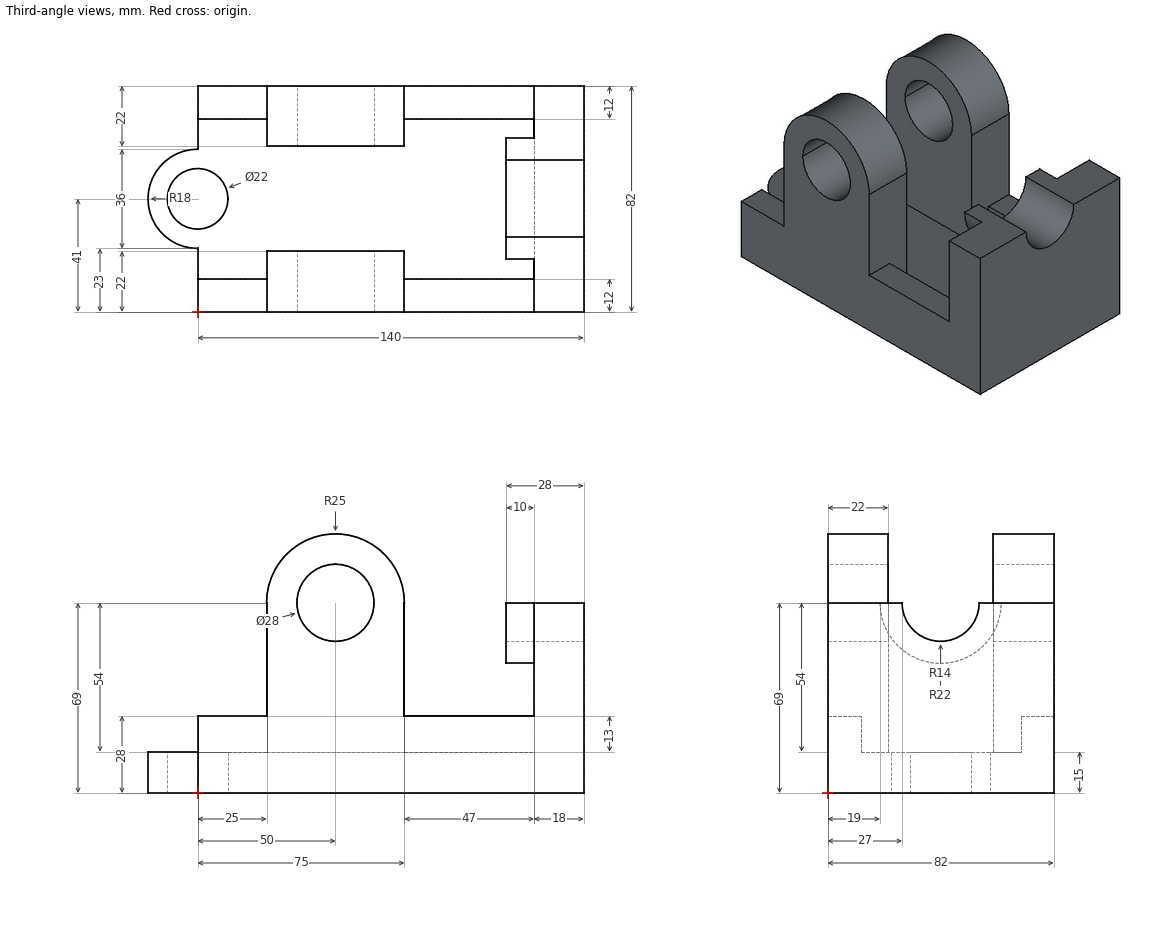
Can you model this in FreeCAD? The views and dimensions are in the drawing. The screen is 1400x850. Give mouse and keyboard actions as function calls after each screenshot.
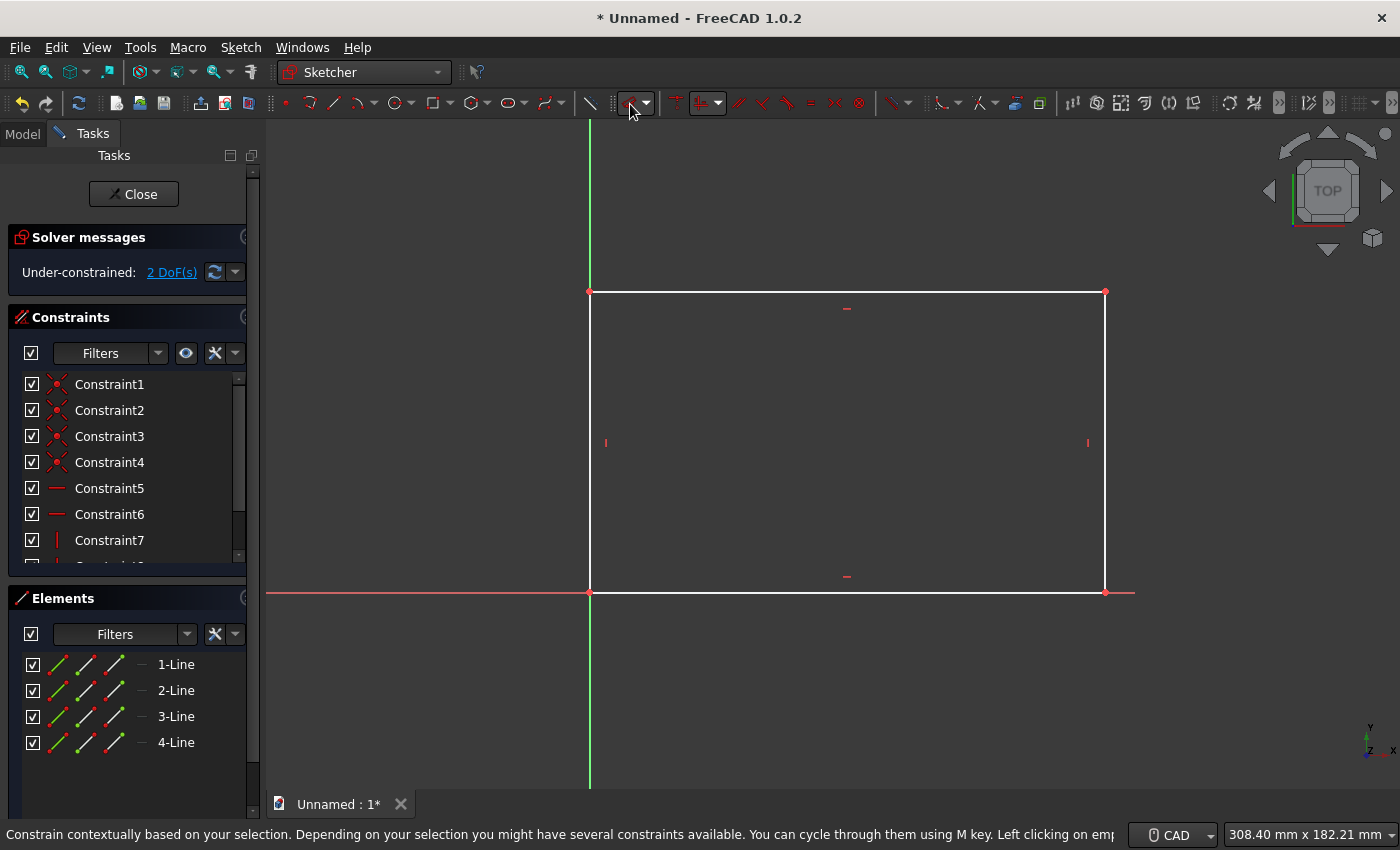
click(1105, 503)
click(1139, 442)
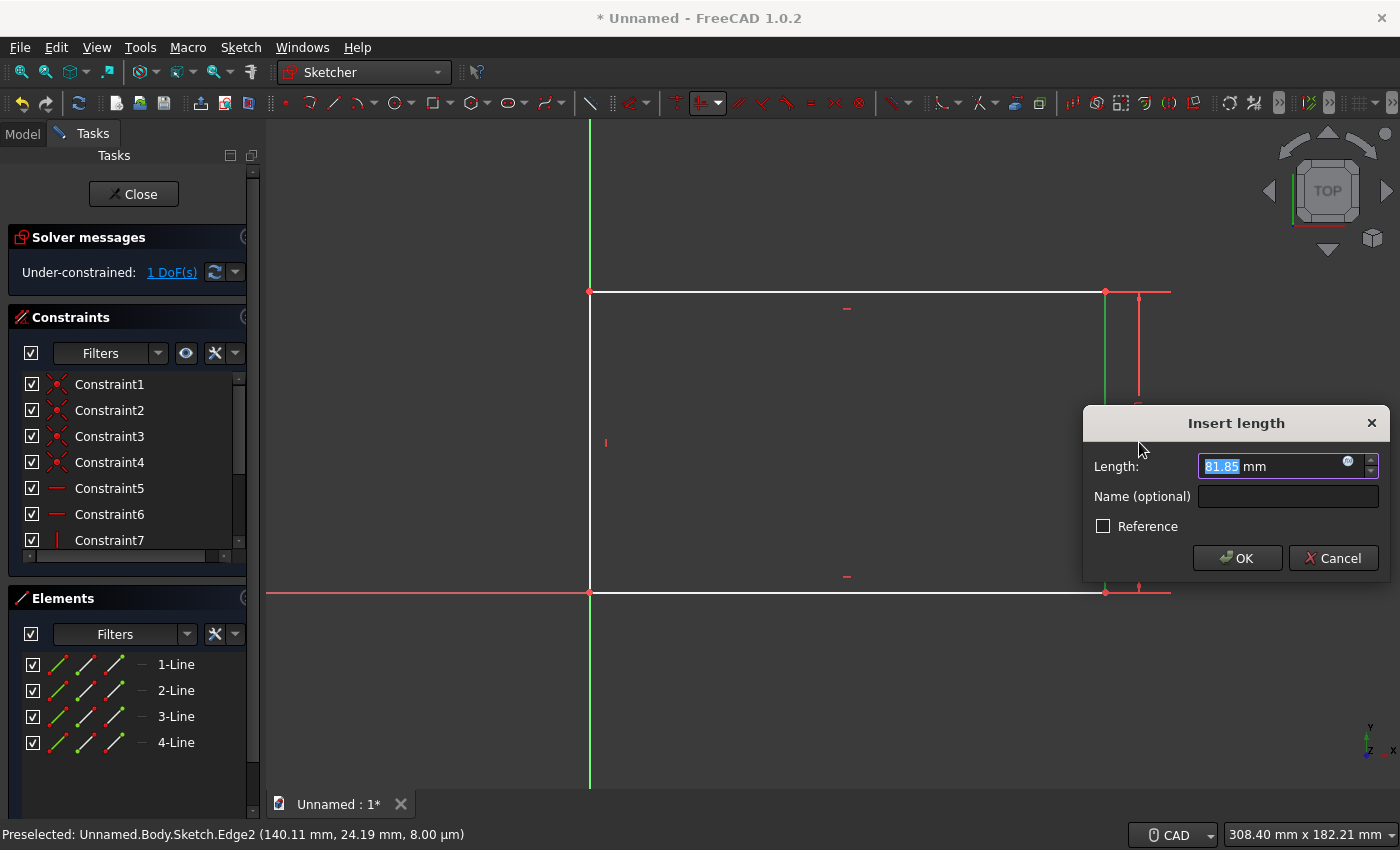
text(82)
key(Return)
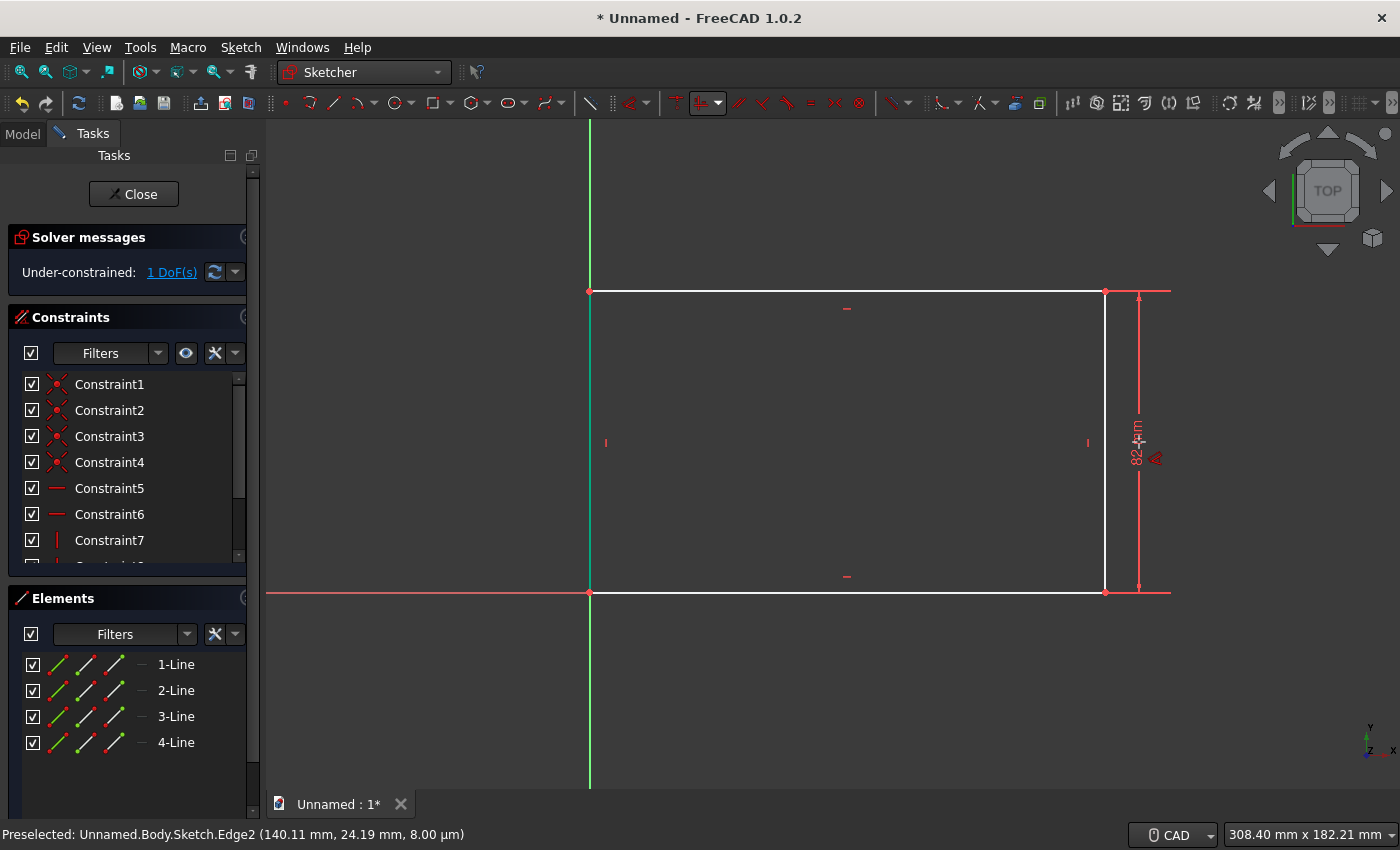
click(744, 593)
click(847, 627)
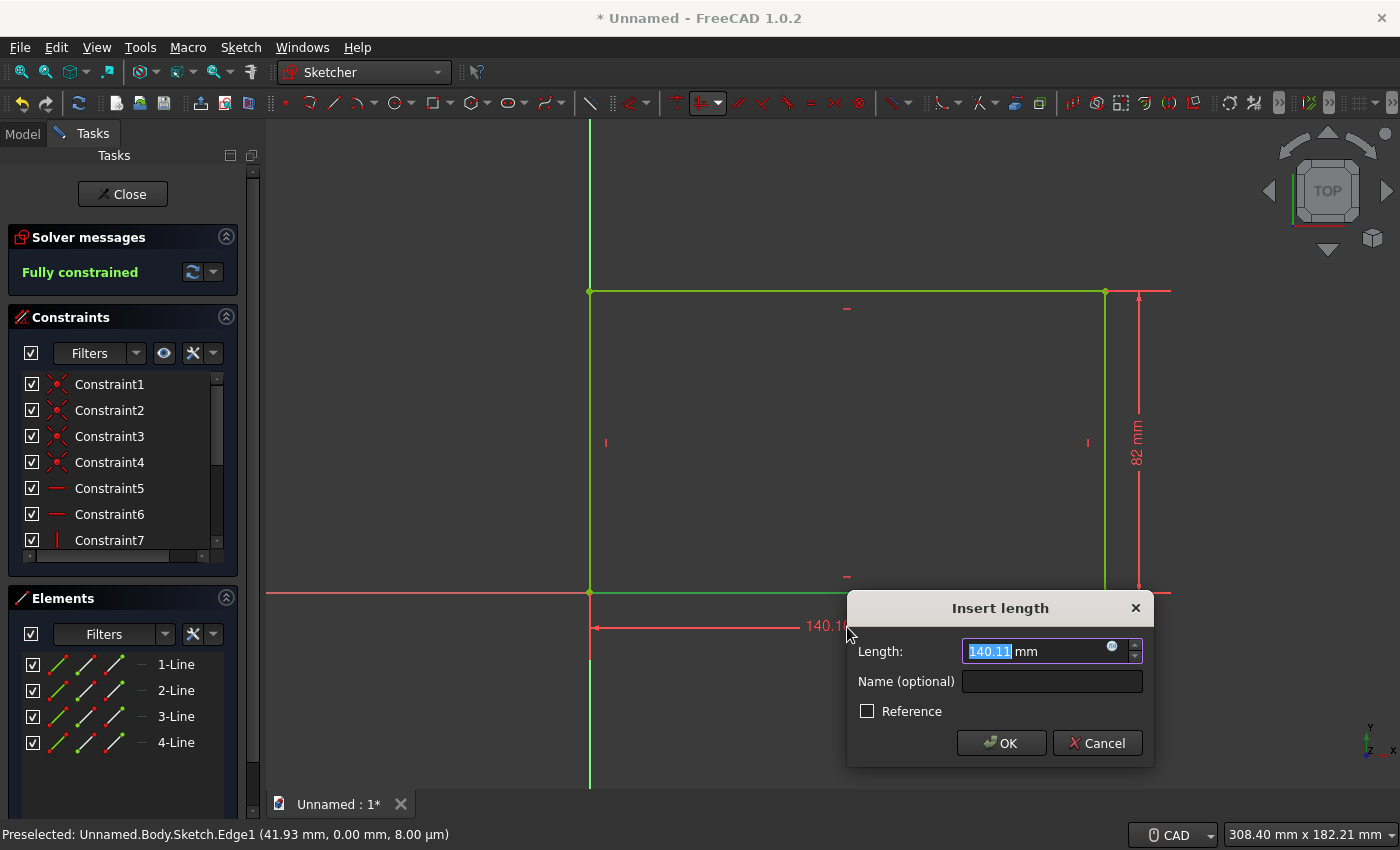
text(140)
key(Return)
key(Escape)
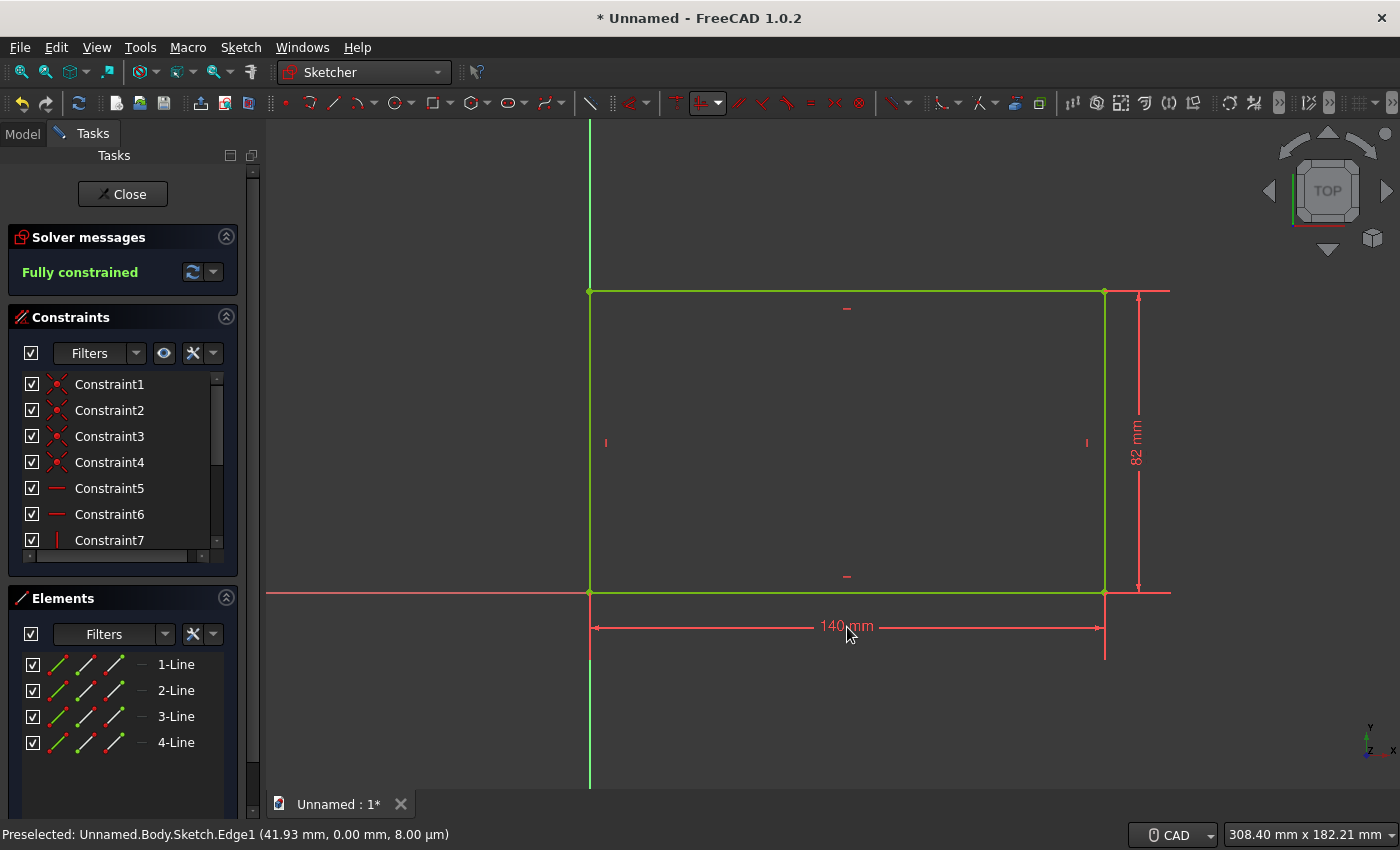
click(123, 194)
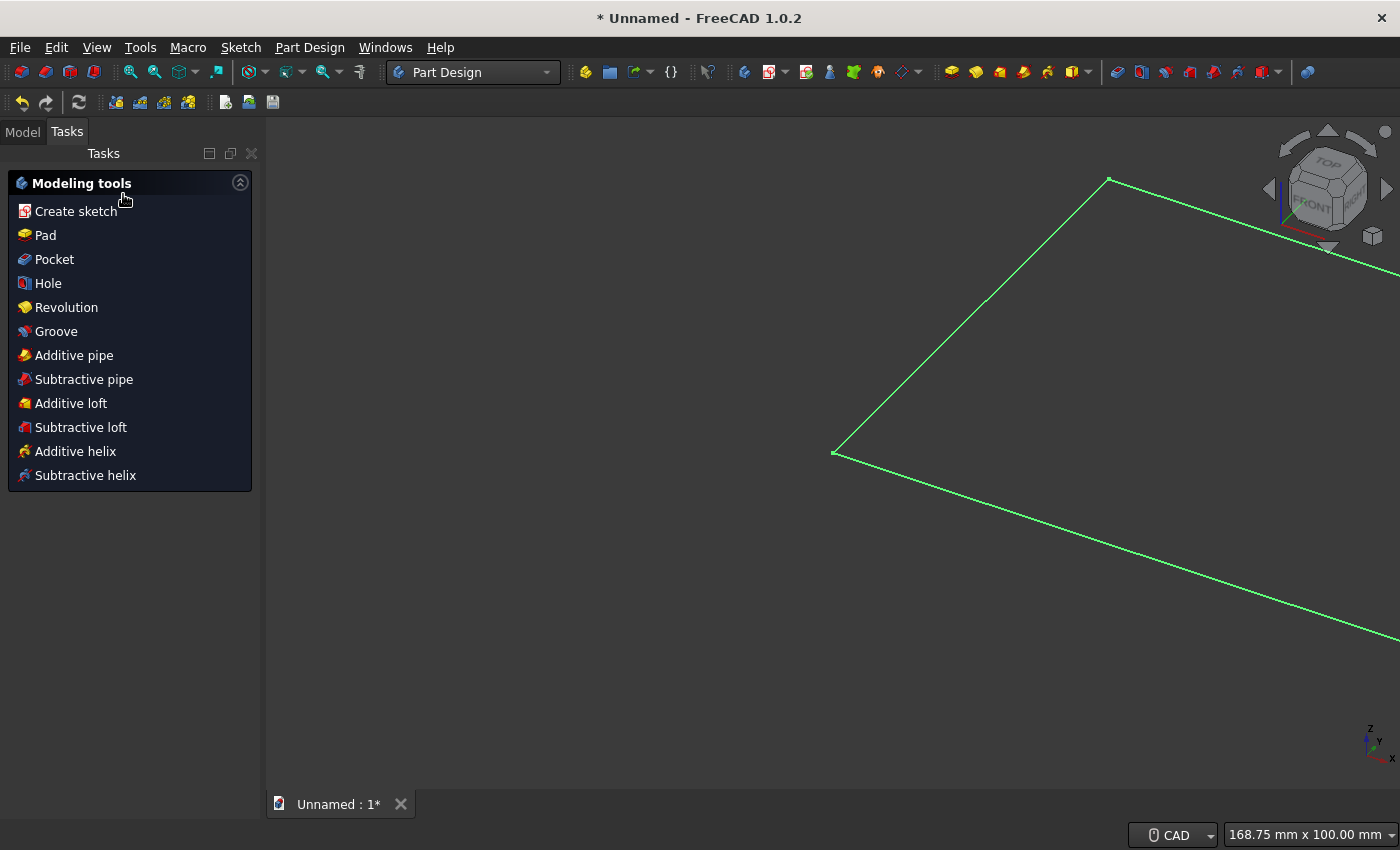
click(952, 72)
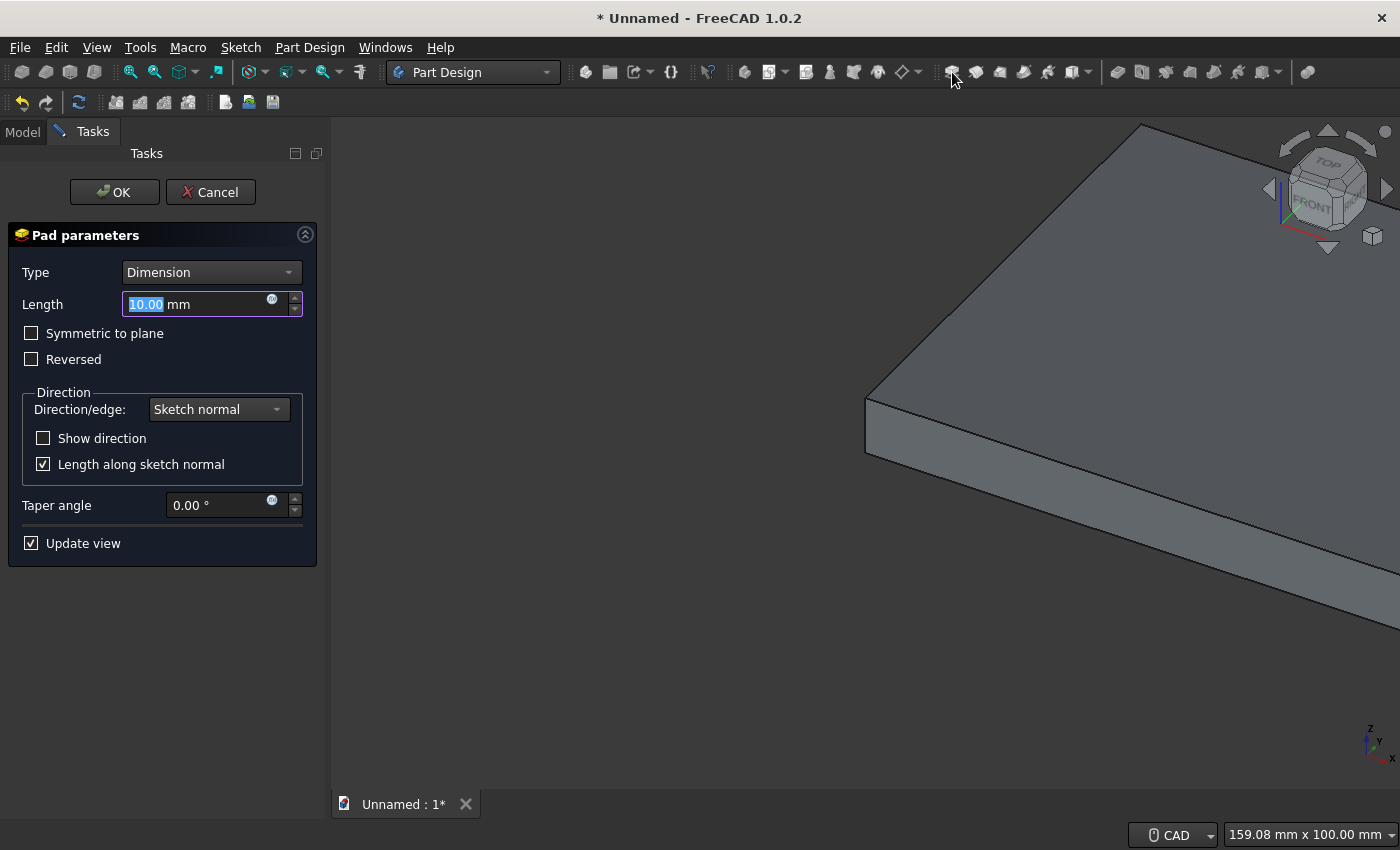
text(15)
key(Tab)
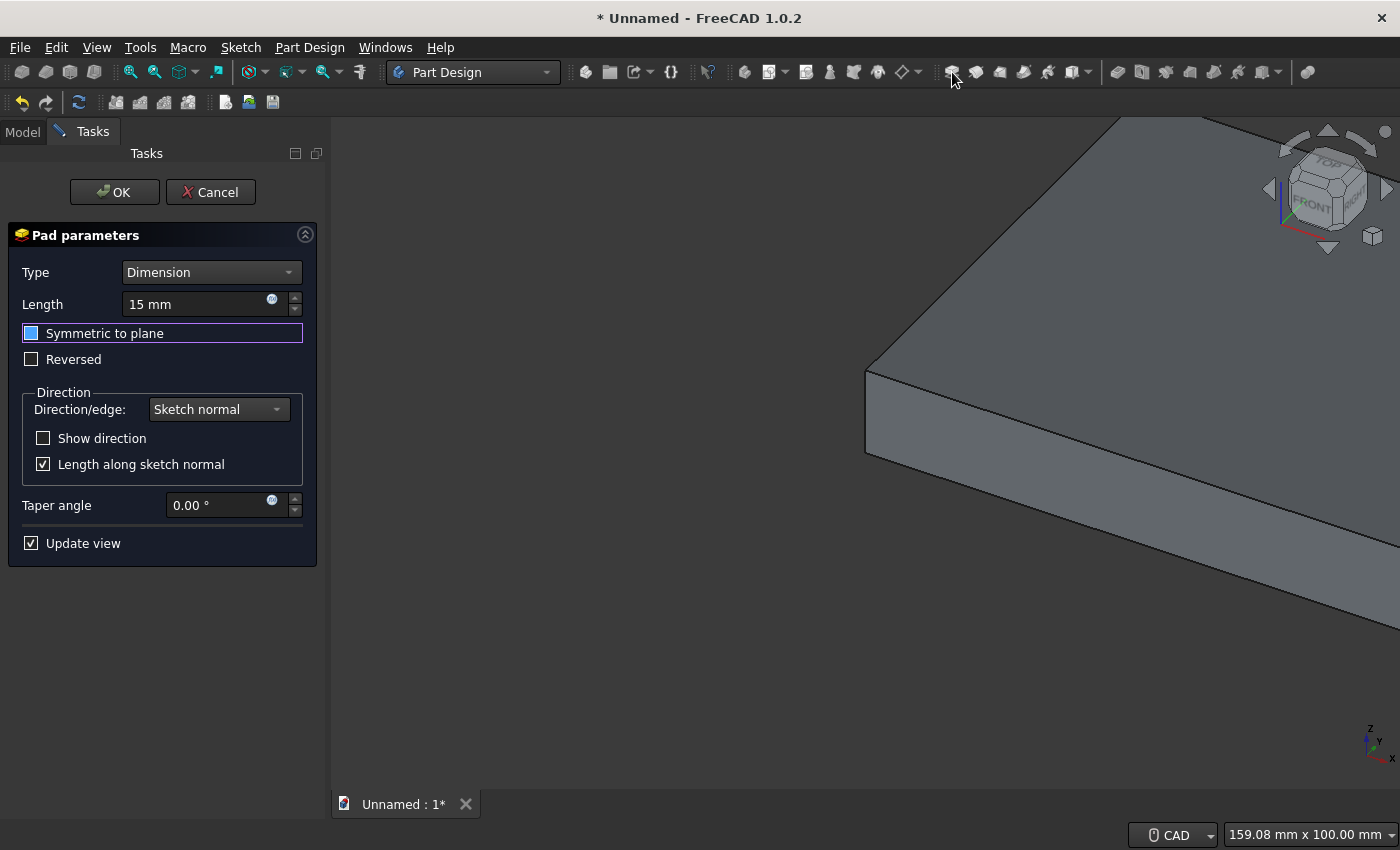
click(115, 192)